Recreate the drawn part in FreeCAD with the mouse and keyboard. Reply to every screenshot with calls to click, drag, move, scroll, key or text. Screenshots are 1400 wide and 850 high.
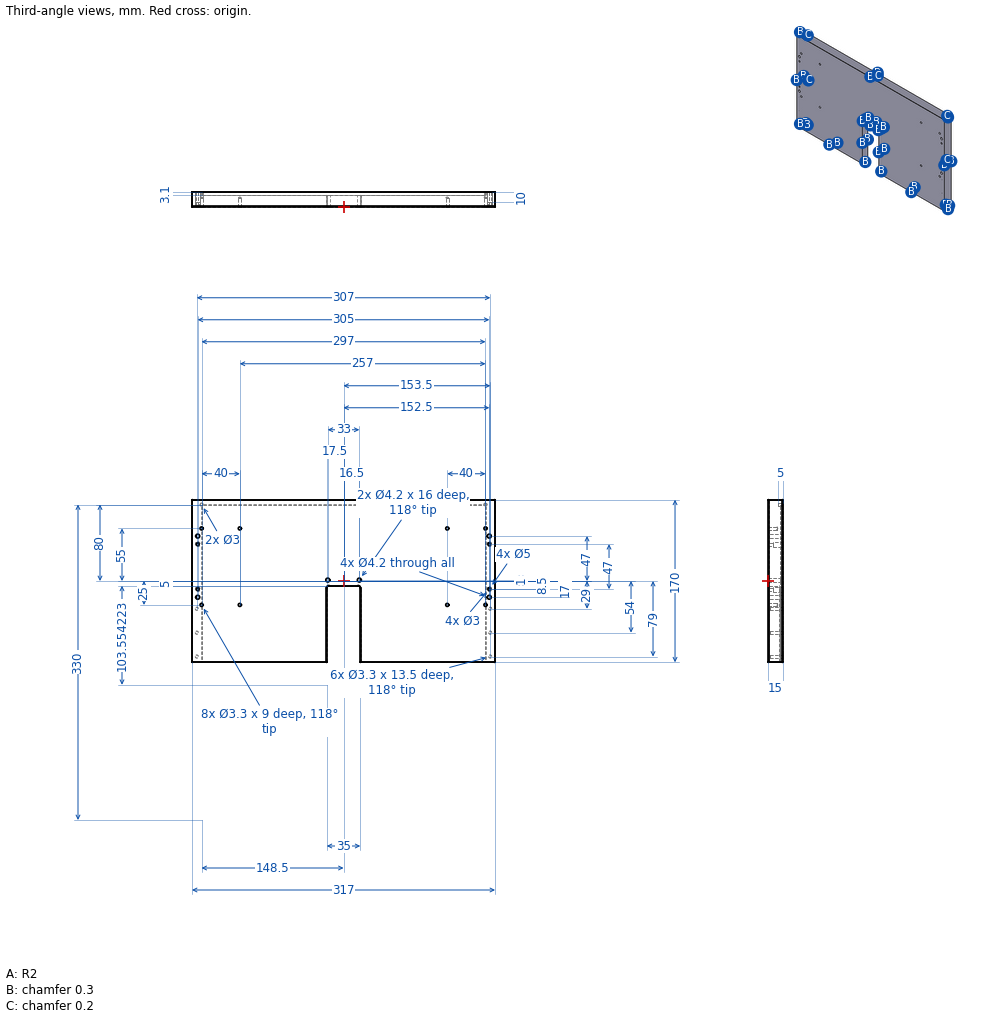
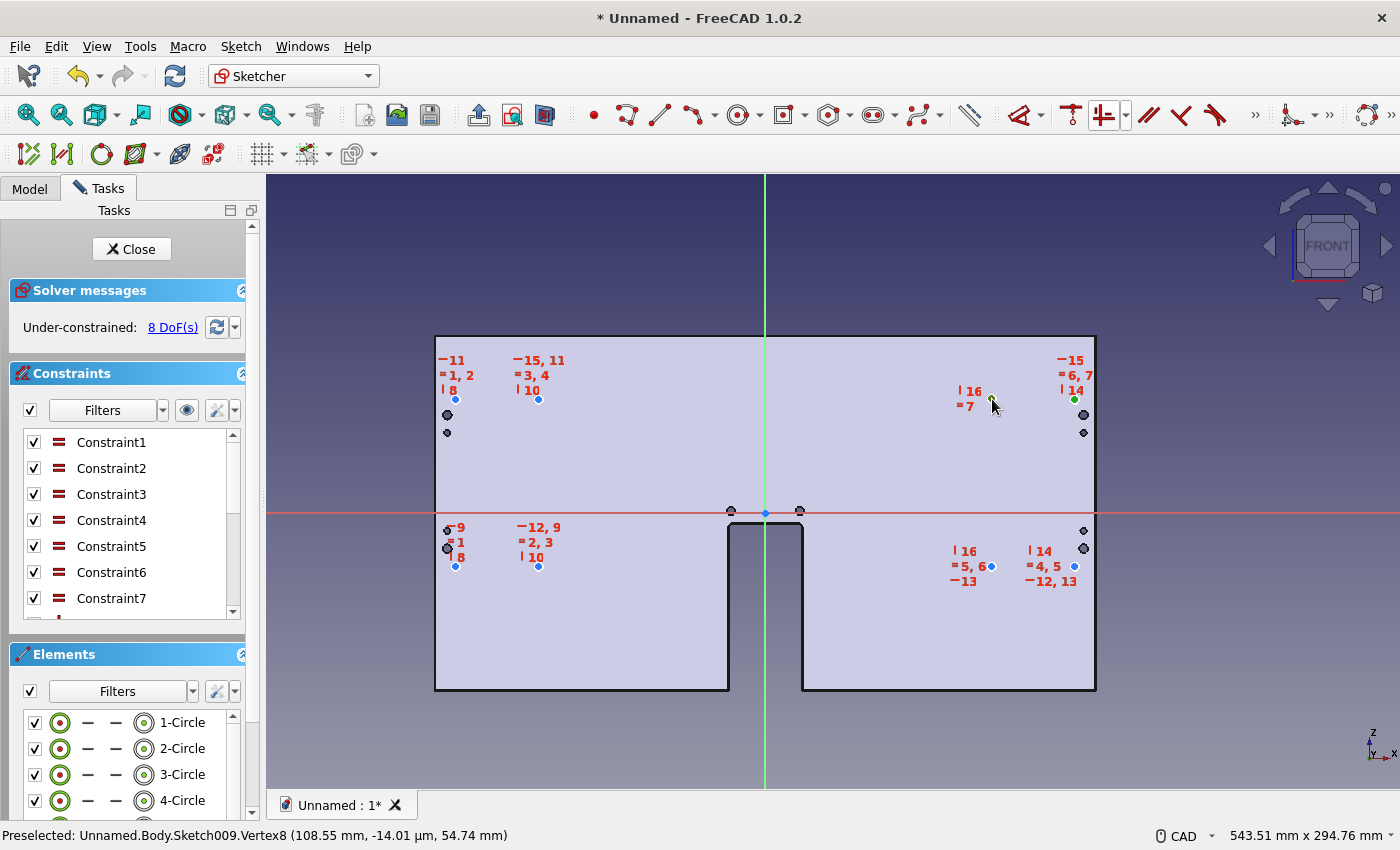
key(h)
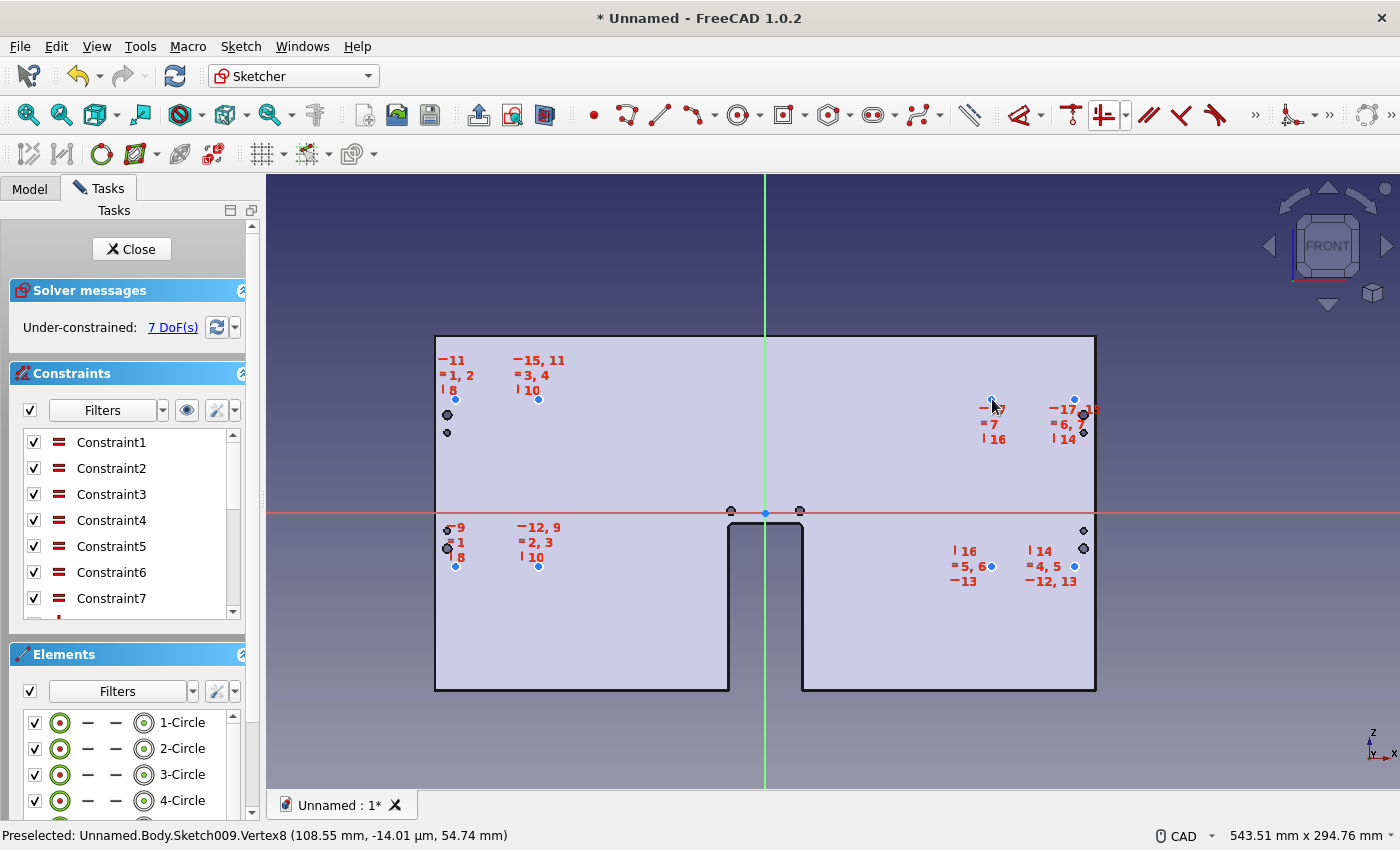
click(1018, 116)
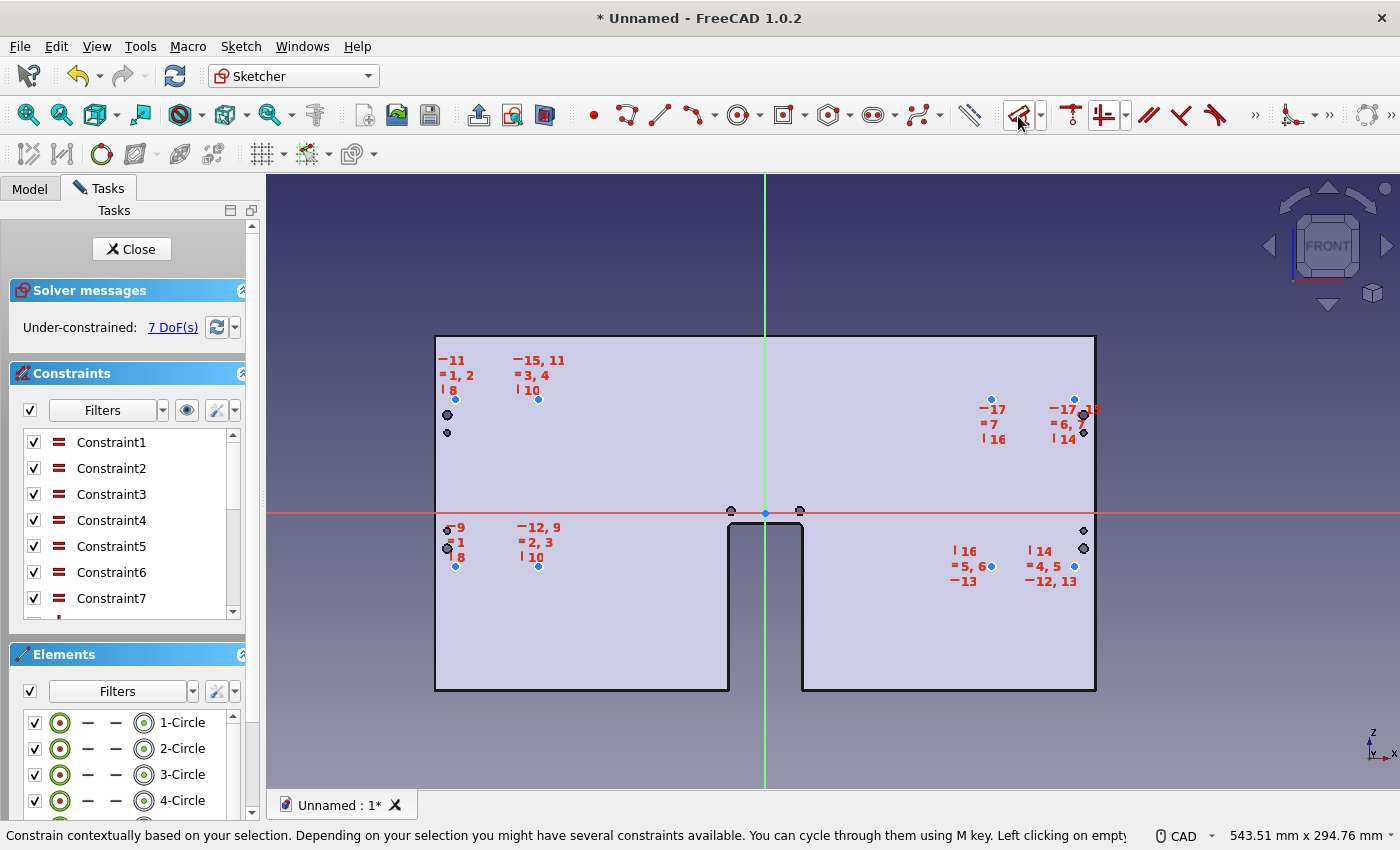
scroll(452, 567, up, 9)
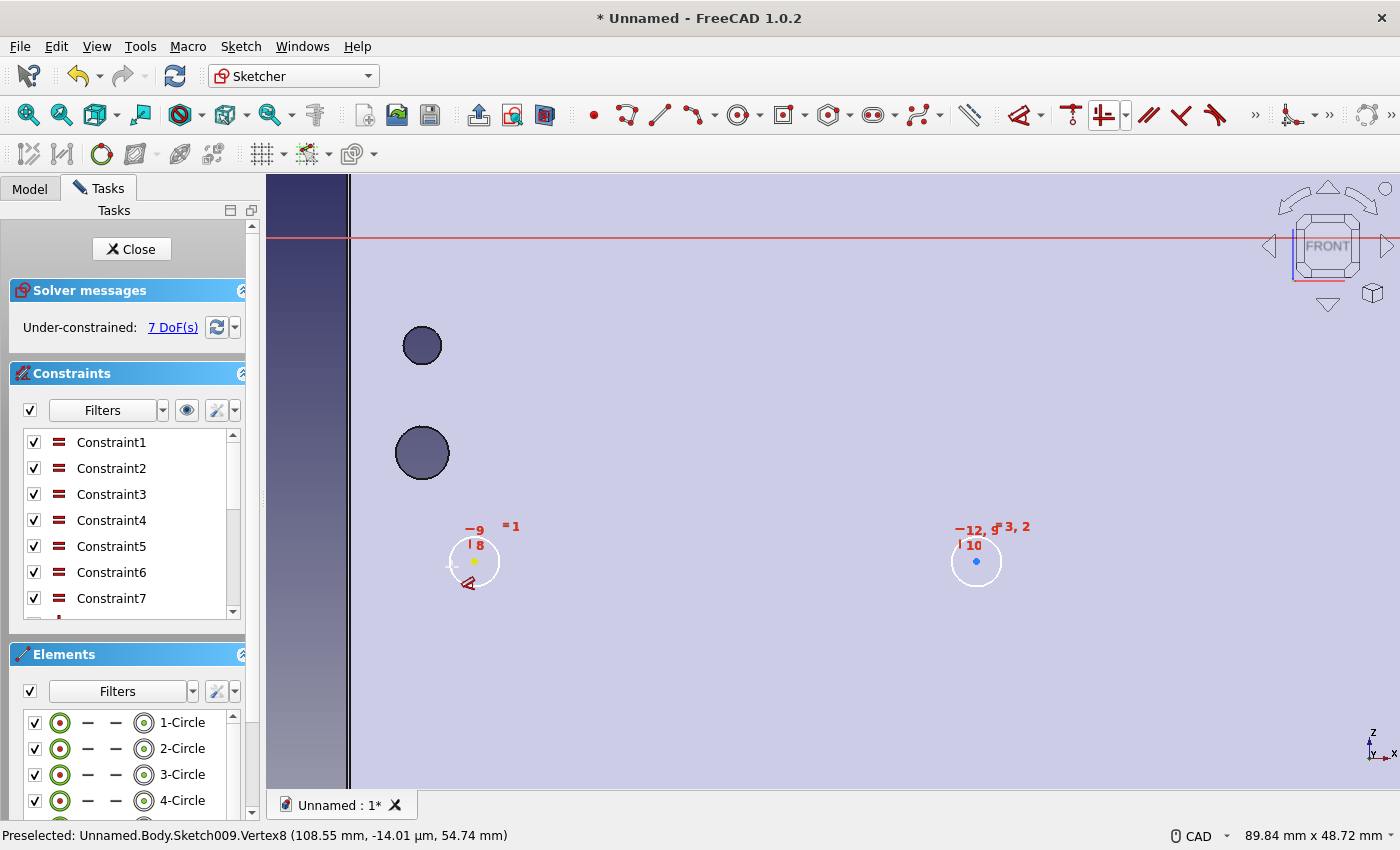
click(450, 561)
click(418, 560)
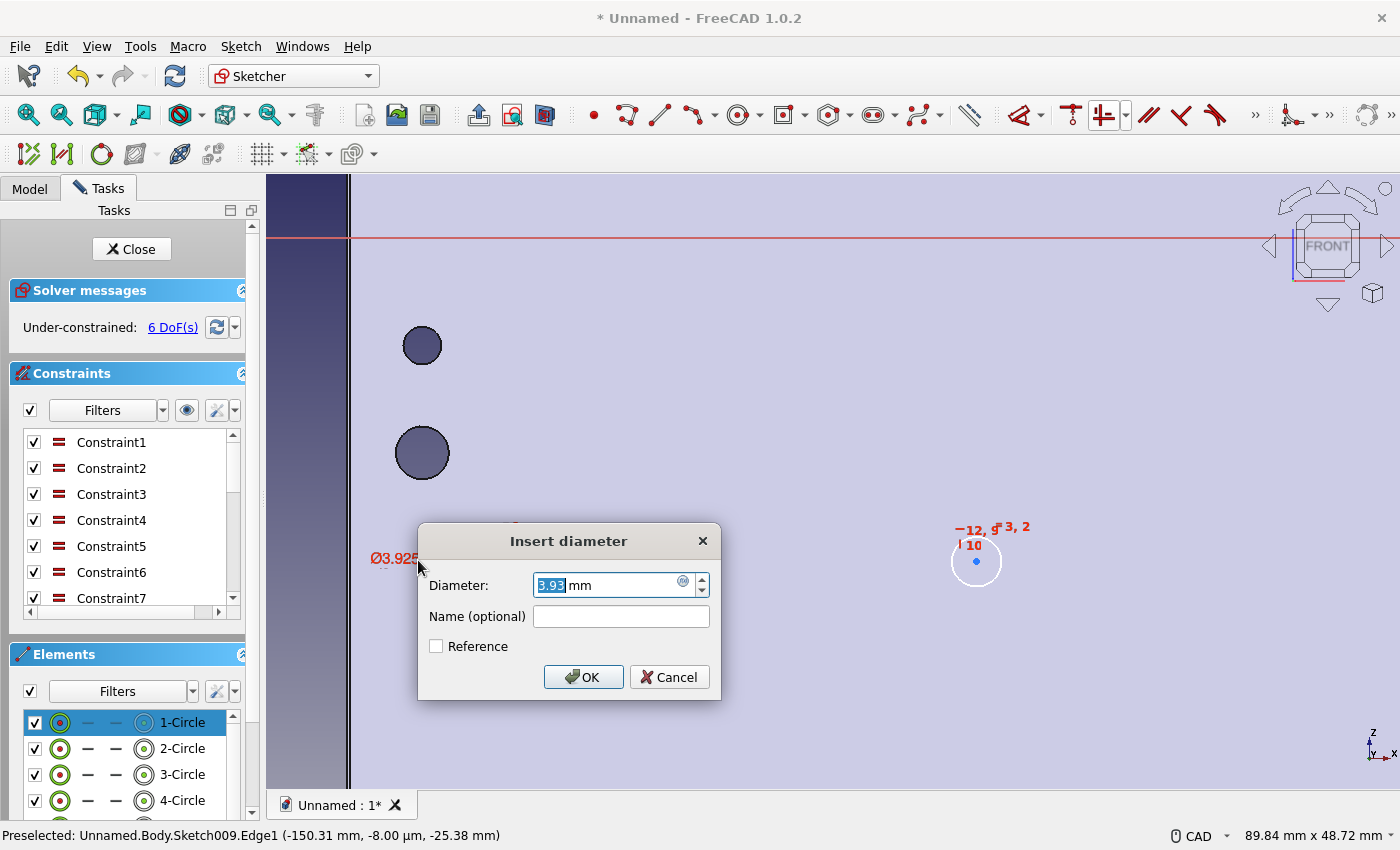
text(3.3)
key(Return)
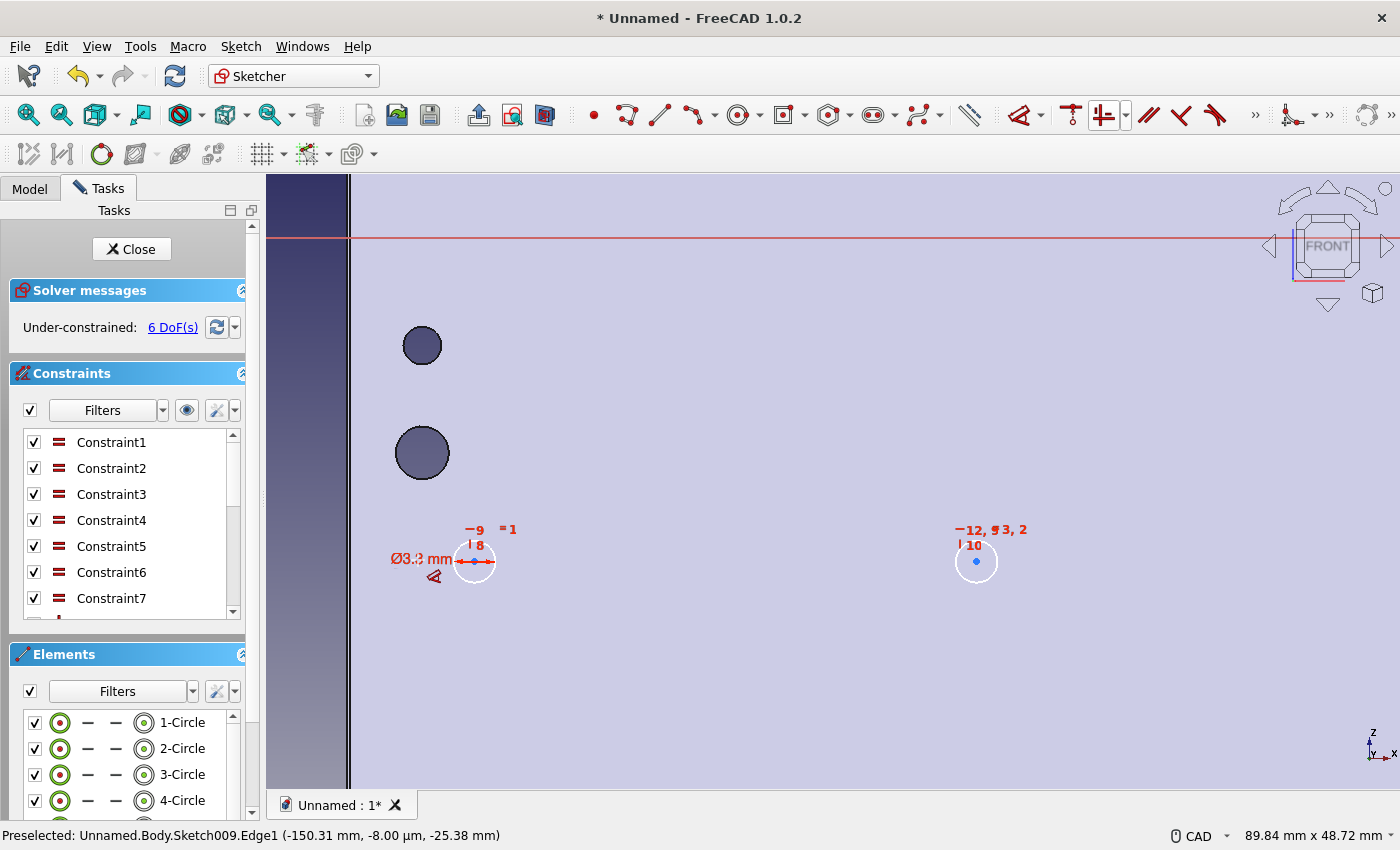
scroll(451, 567, down, 9)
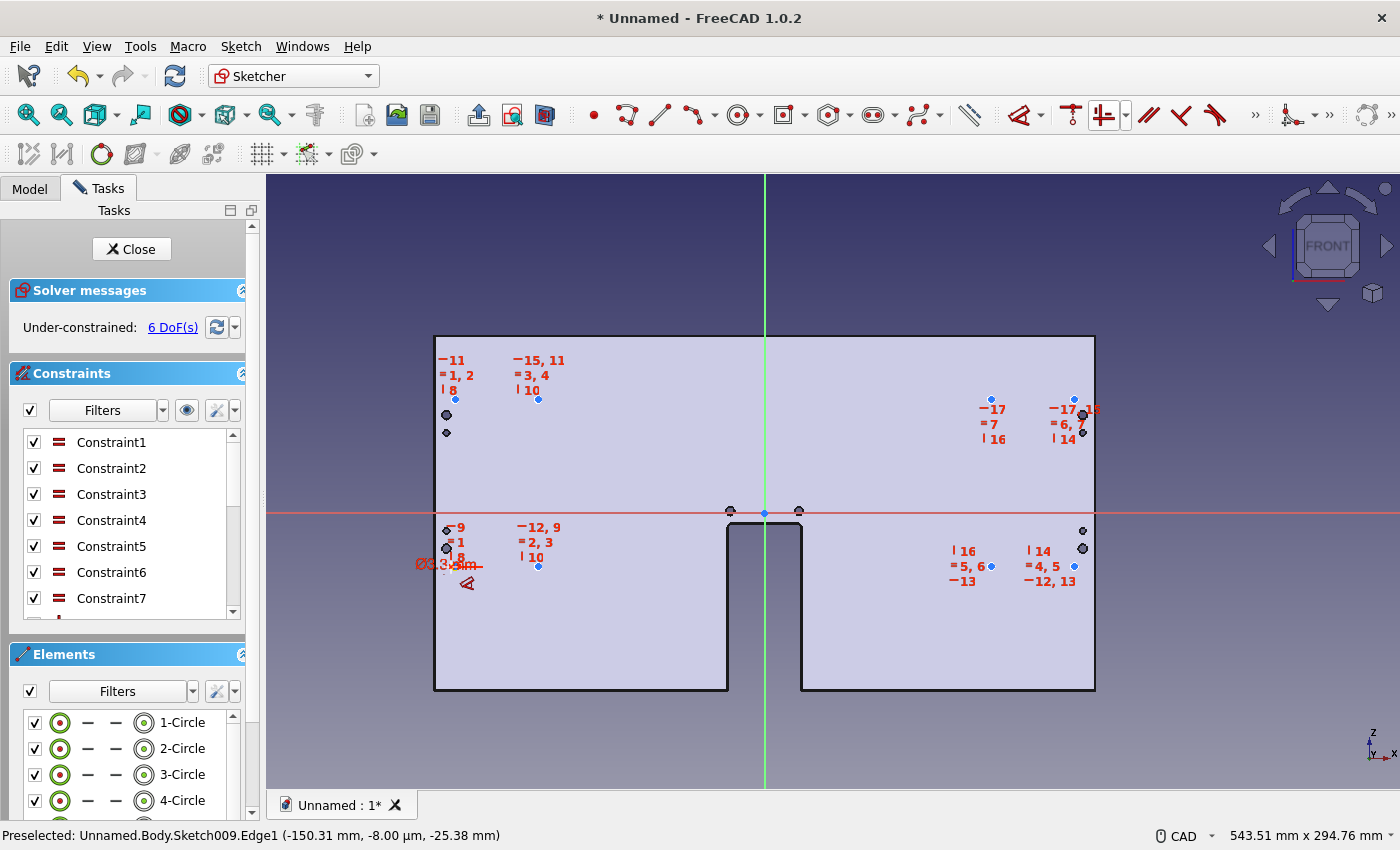
click(455, 567)
click(421, 540)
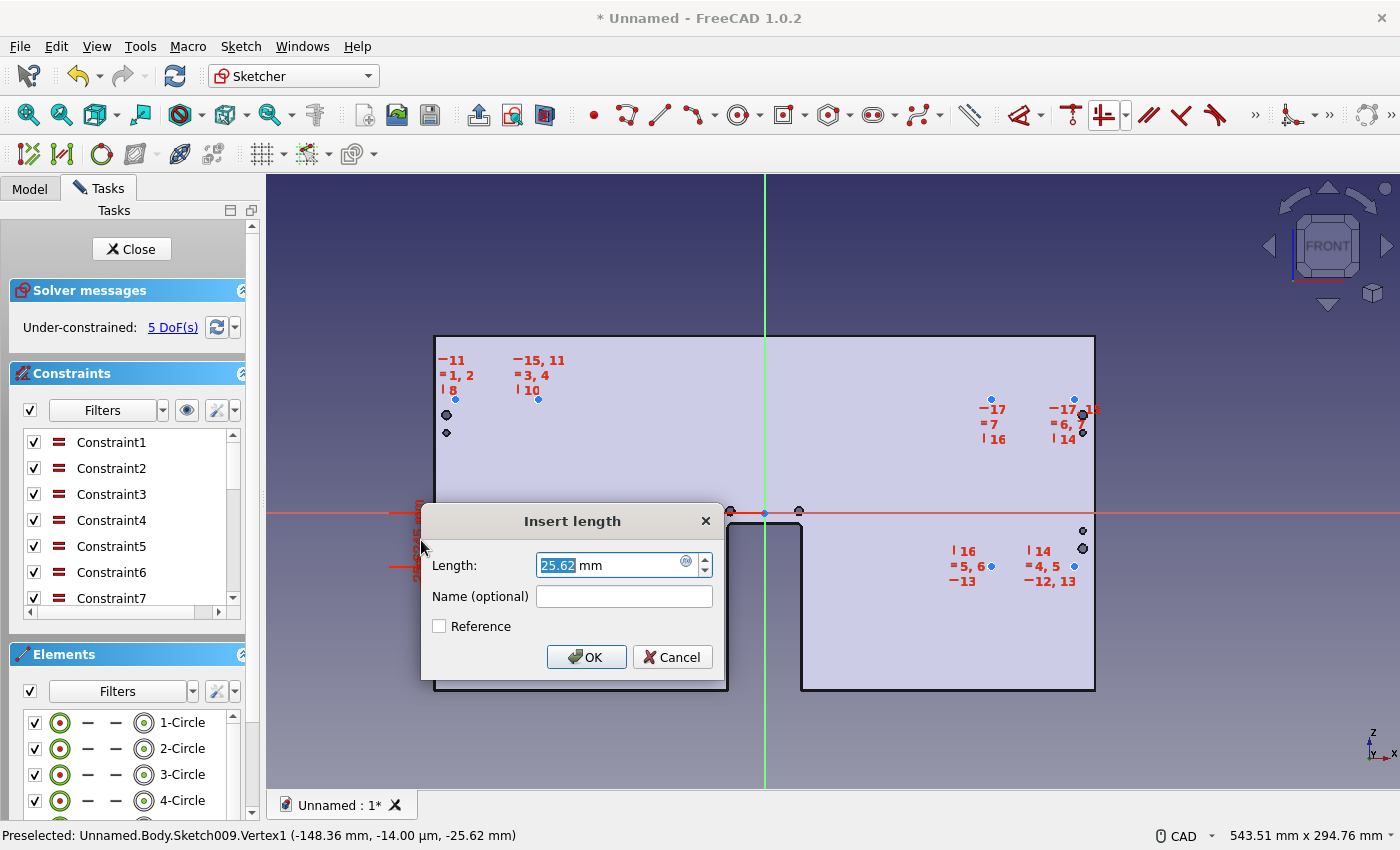
text(25)
key(Return)